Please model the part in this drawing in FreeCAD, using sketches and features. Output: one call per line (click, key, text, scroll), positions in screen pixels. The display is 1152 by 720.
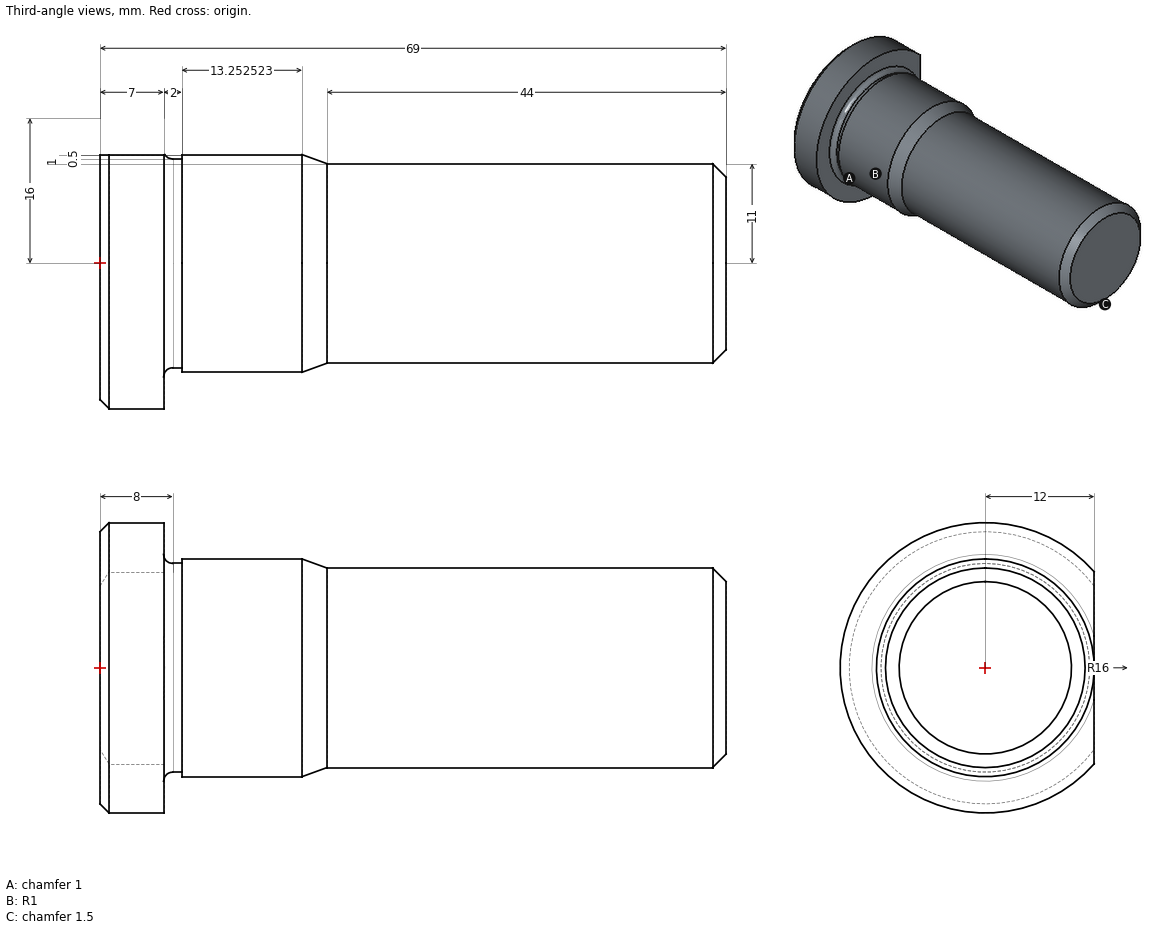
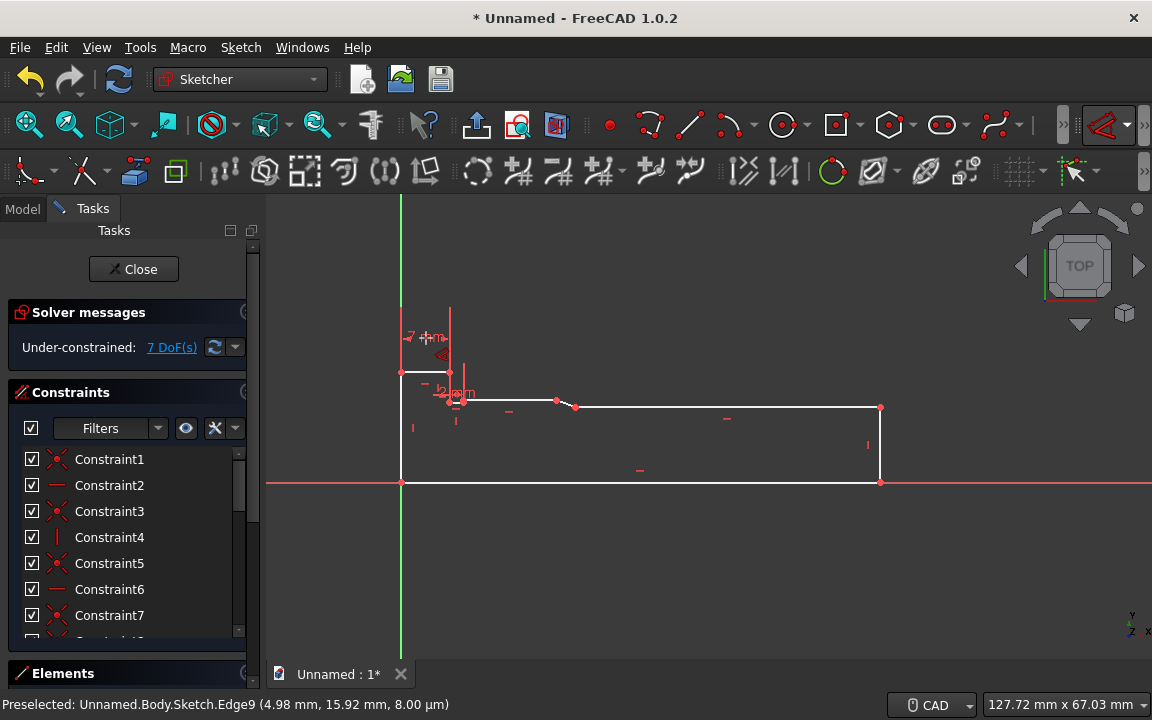
click(545, 483)
click(641, 517)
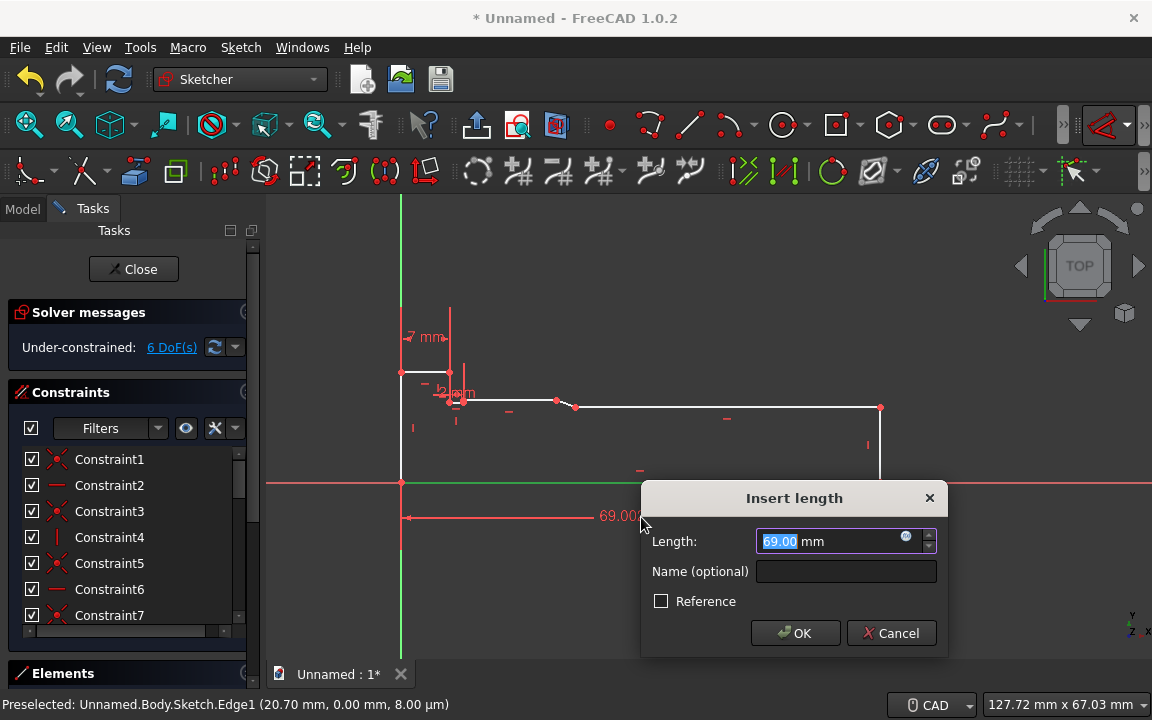
text(69)
key(Return)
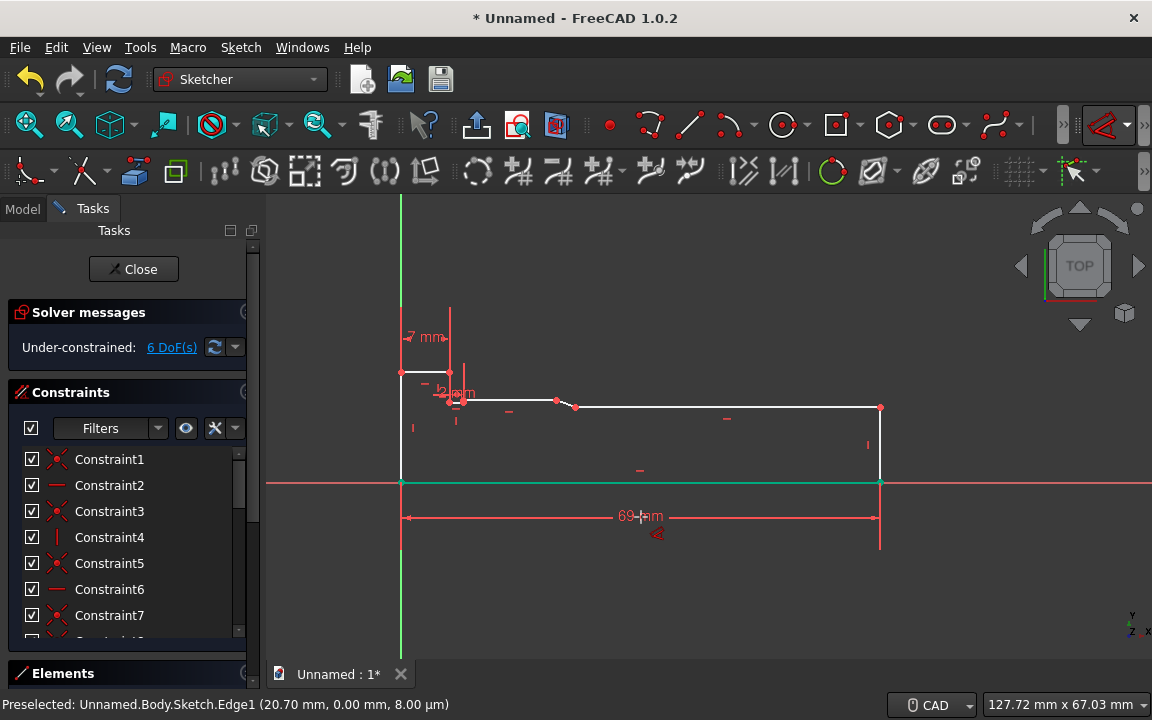
click(880, 460)
click(914, 445)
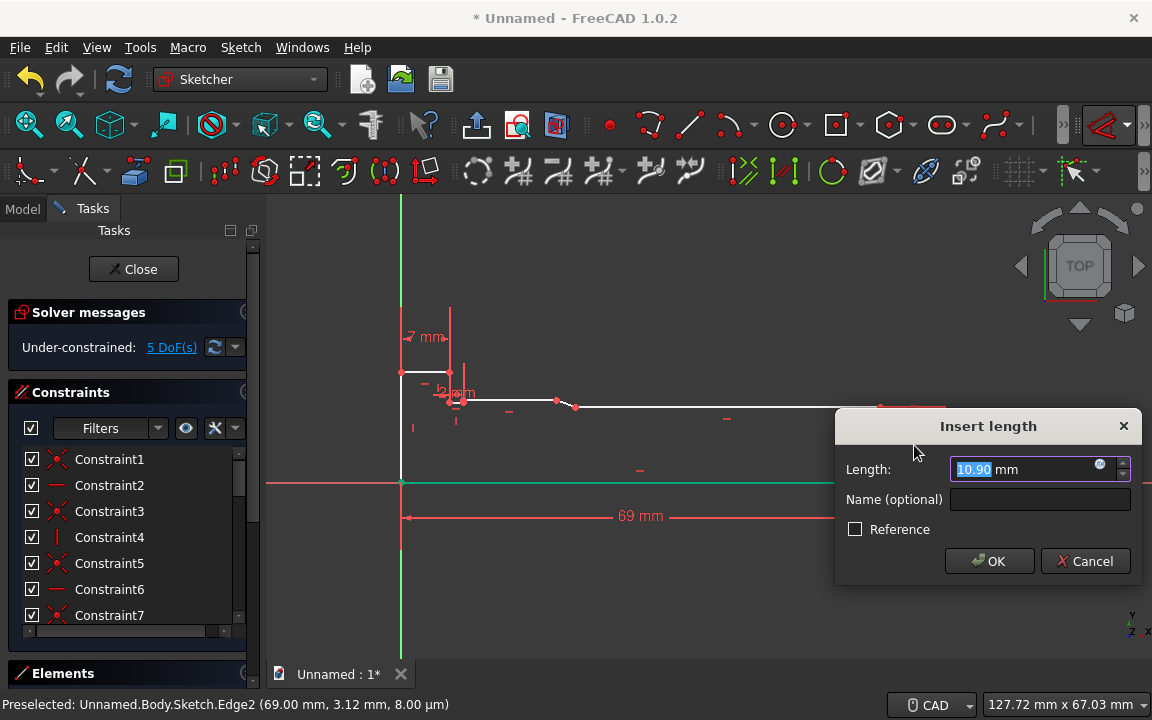
text(11)
key(Return)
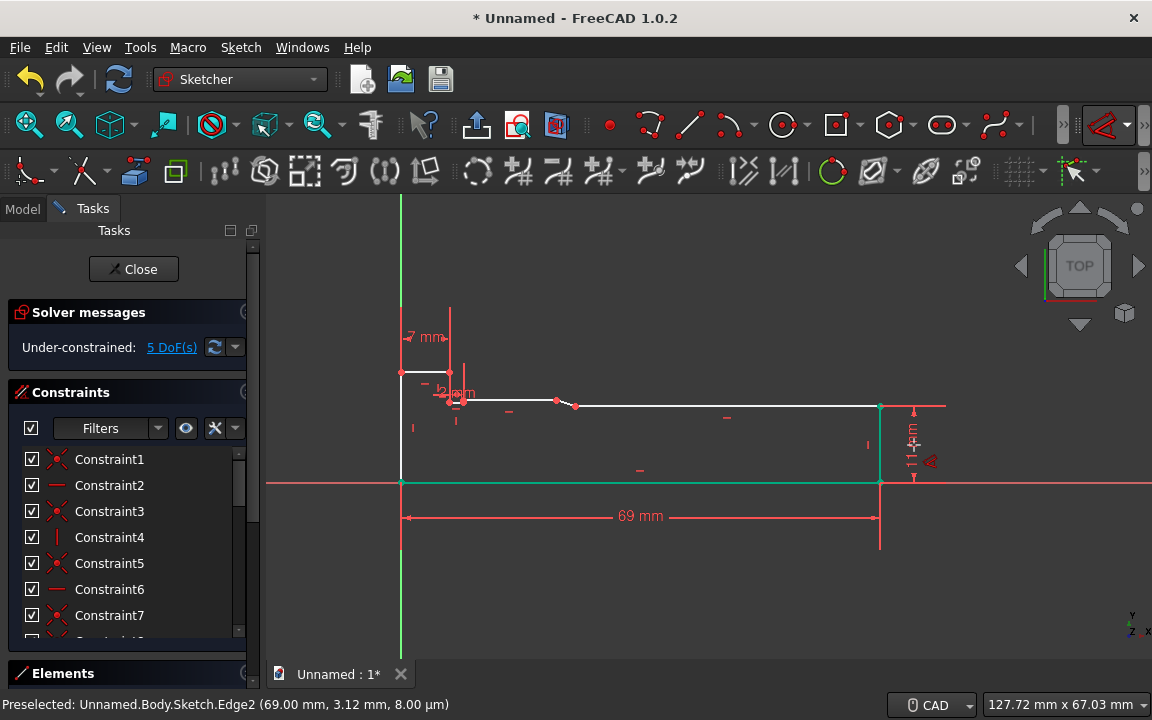
click(789, 406)
click(728, 372)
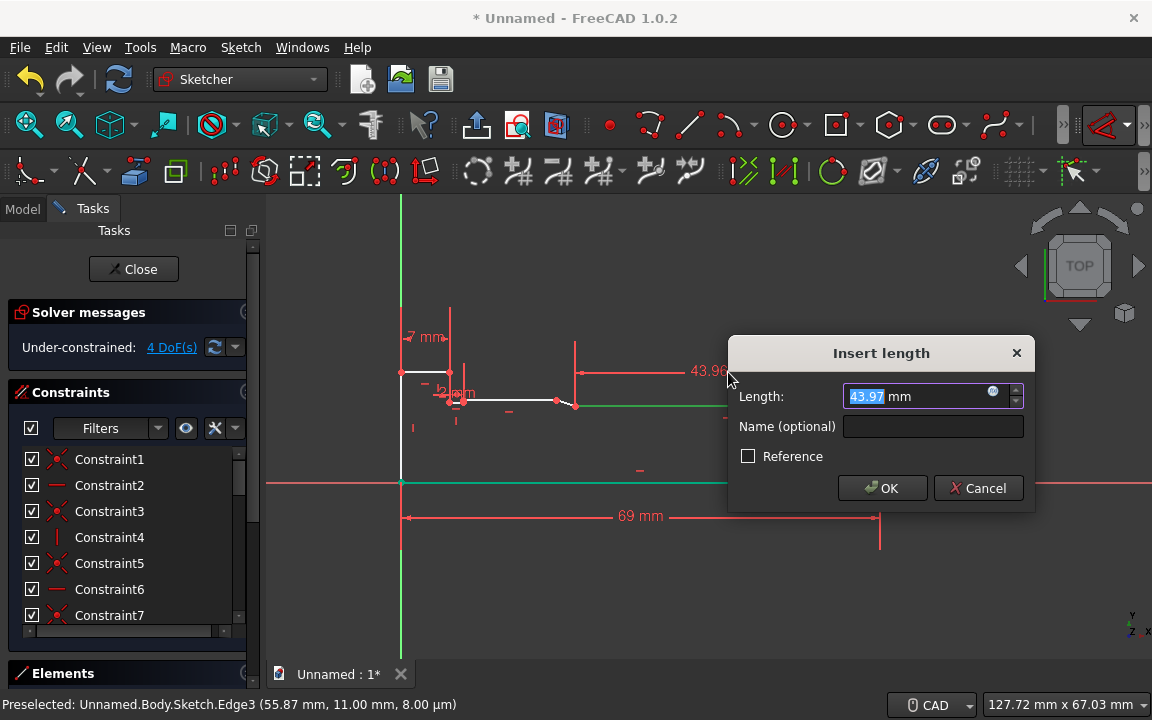
text(44)
key(Return)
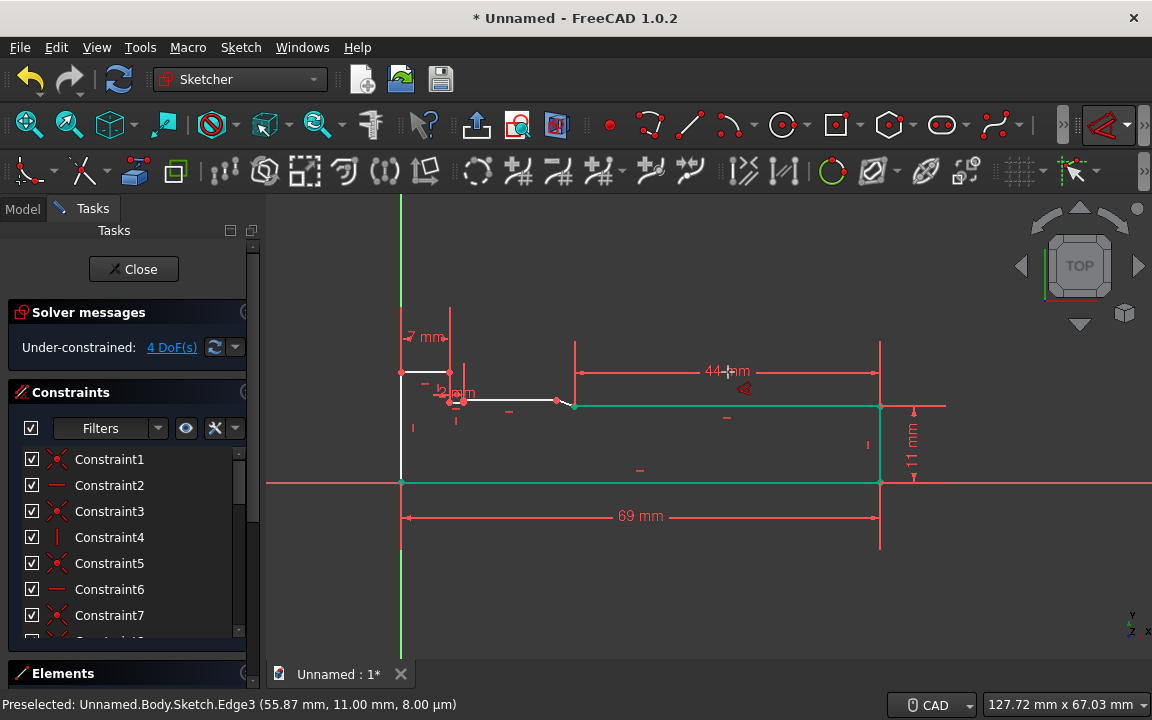
click(401, 405)
click(367, 427)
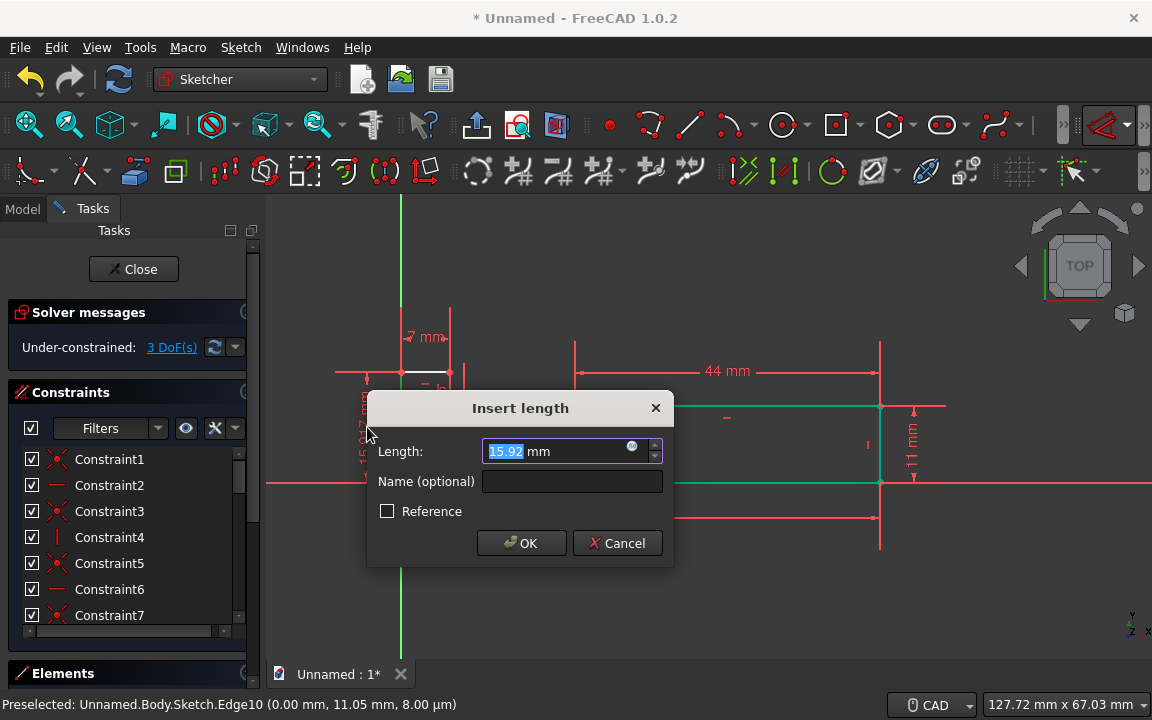
text(16)
key(Return)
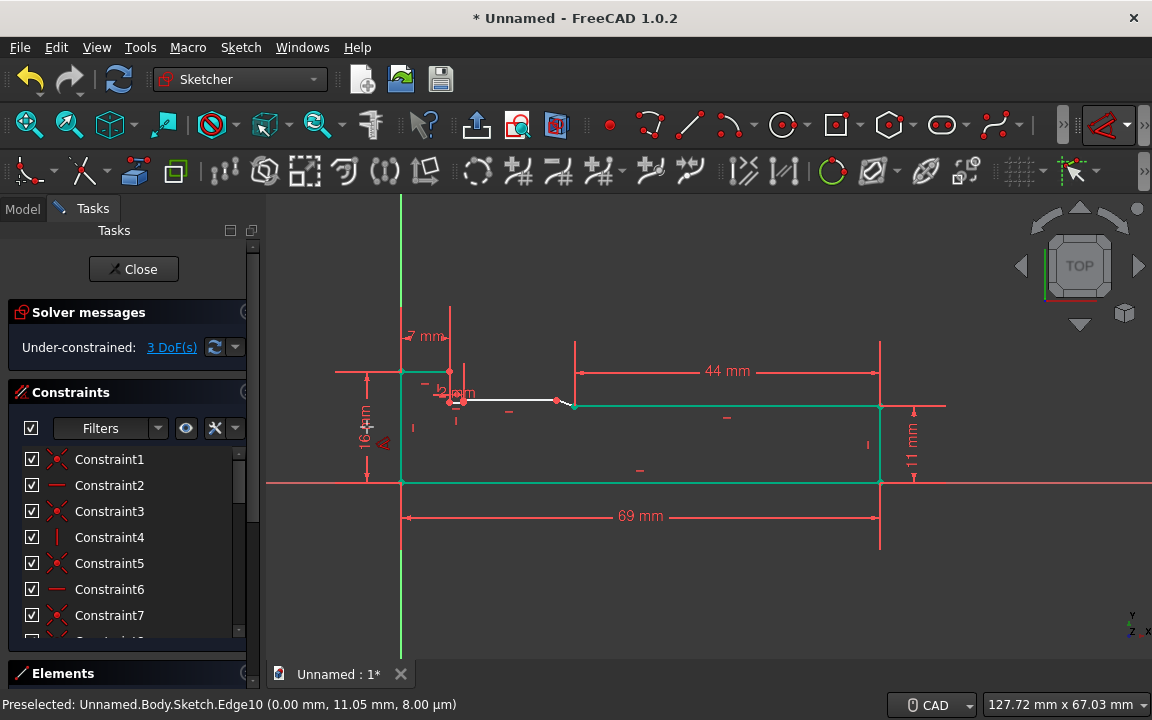
scroll(565, 403, up, 9)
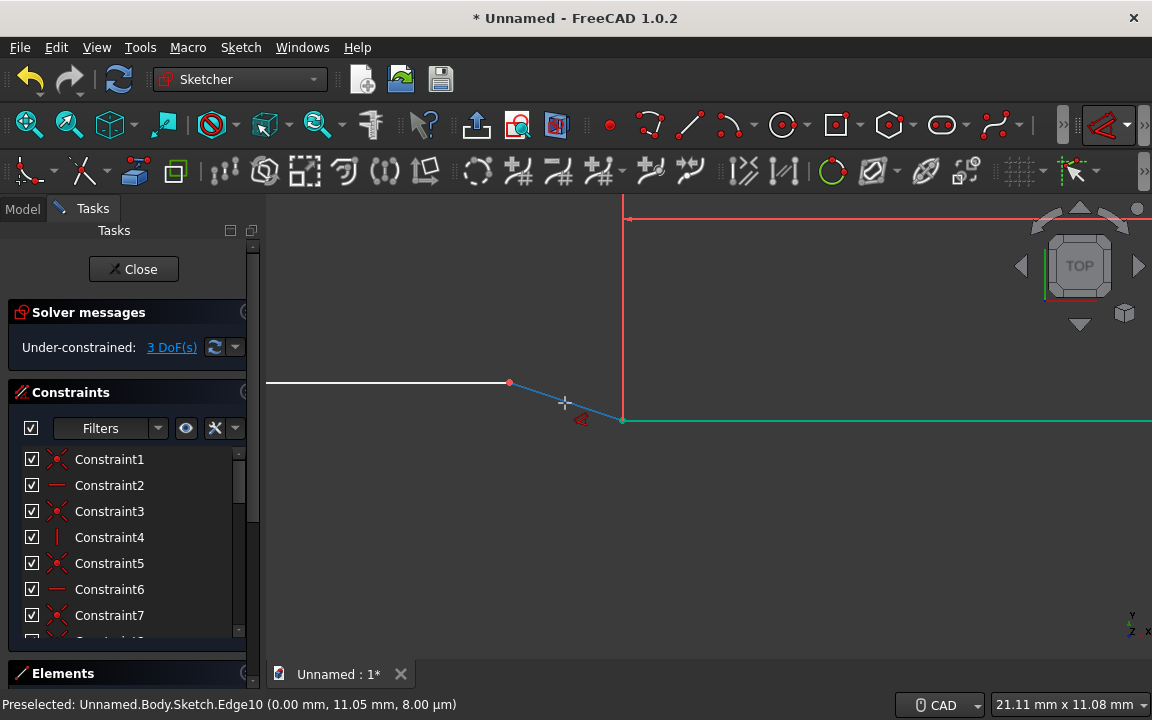
click(566, 402)
click(475, 402)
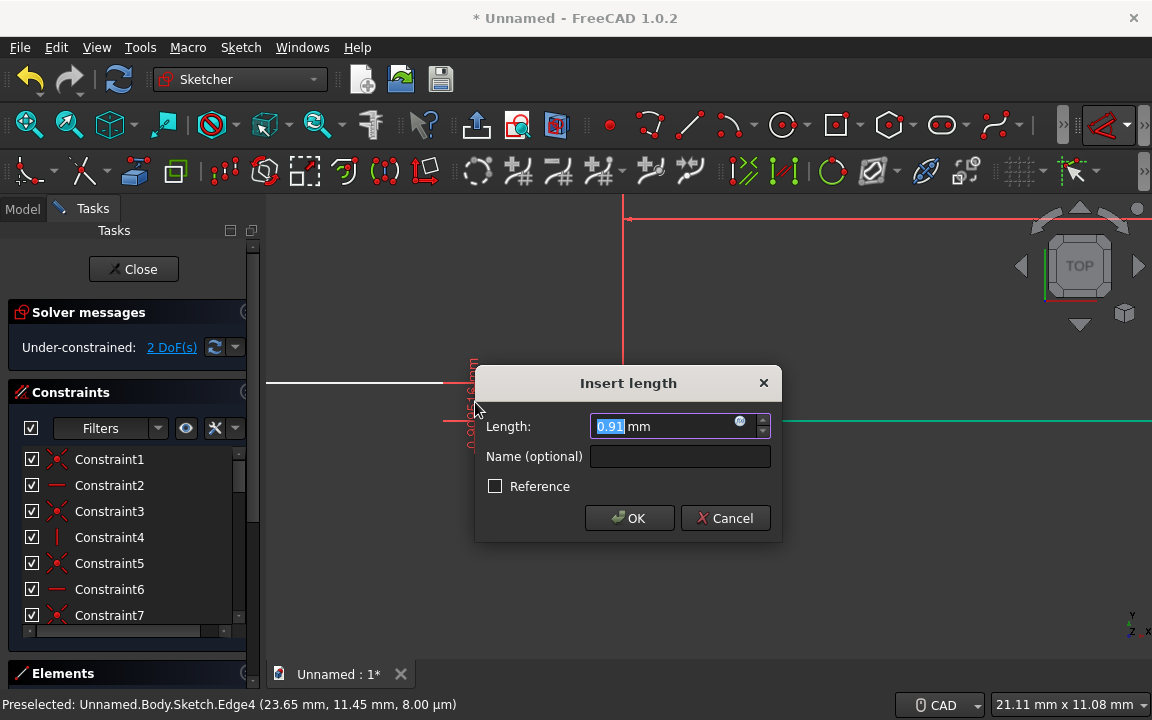
text(1)
key(Return)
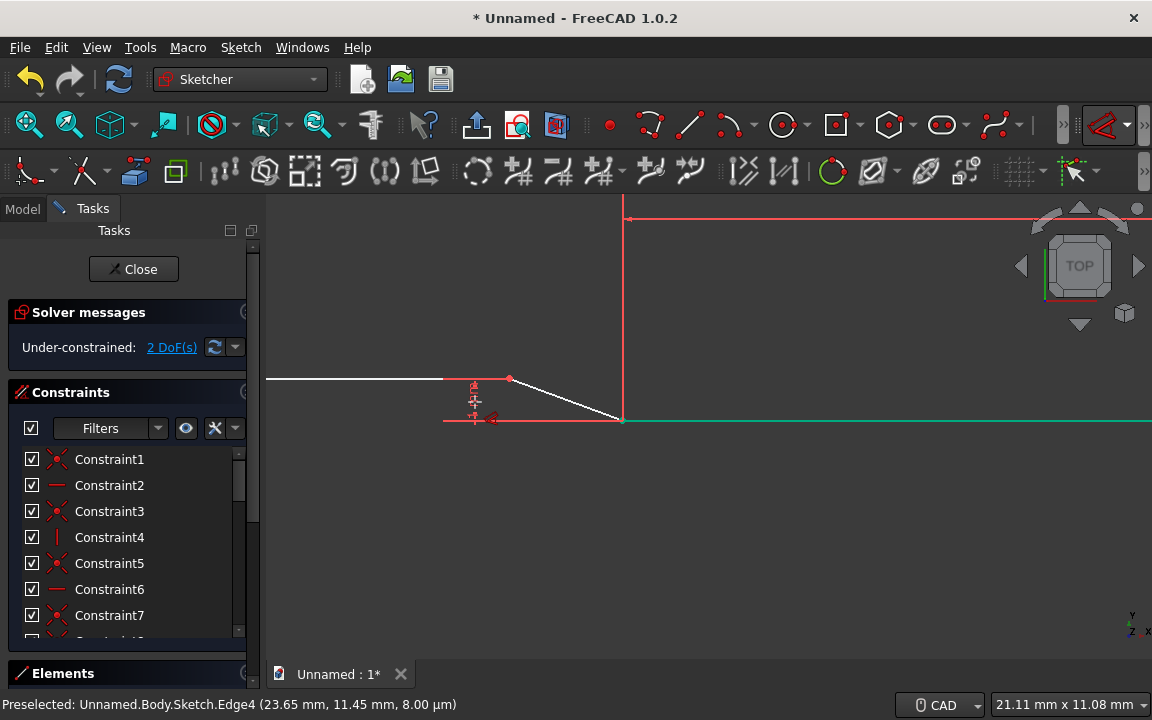
scroll(565, 403, down, 9)